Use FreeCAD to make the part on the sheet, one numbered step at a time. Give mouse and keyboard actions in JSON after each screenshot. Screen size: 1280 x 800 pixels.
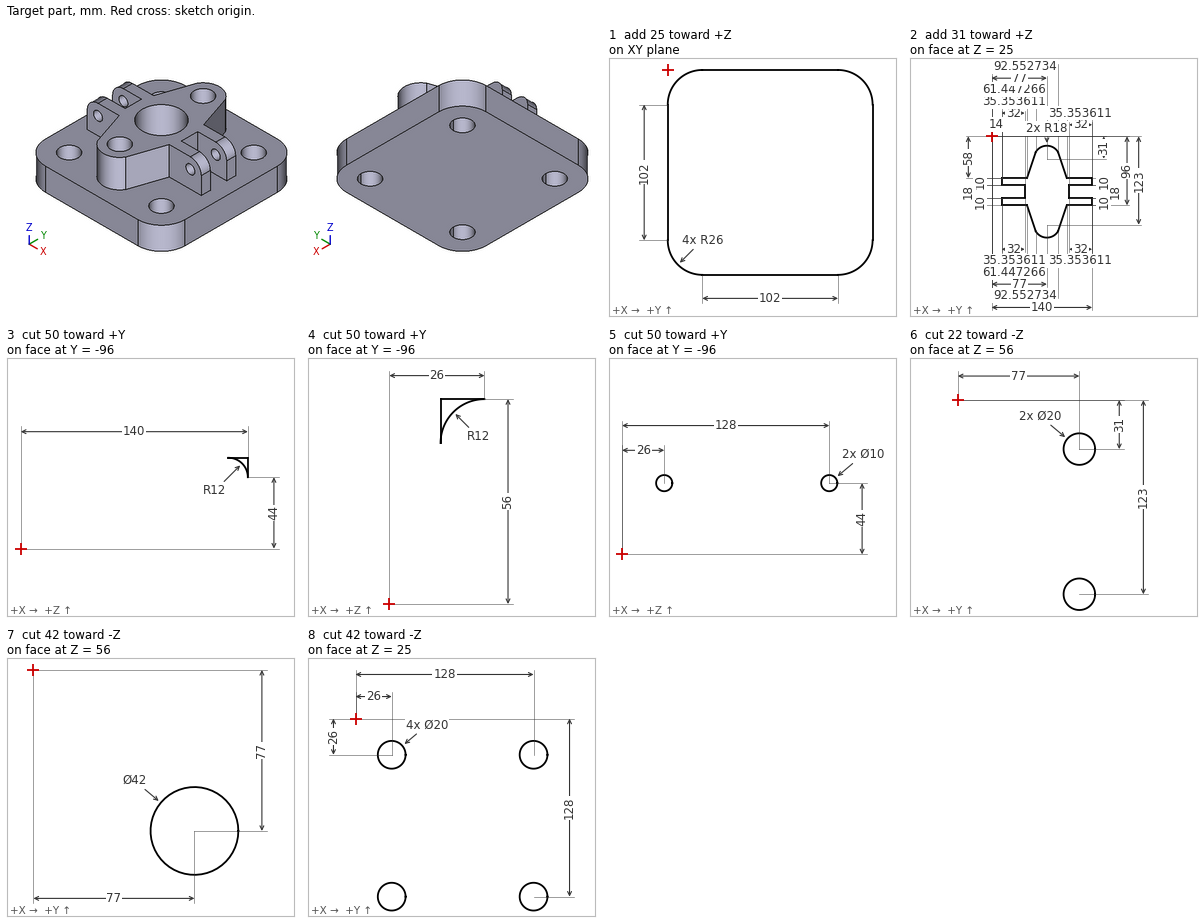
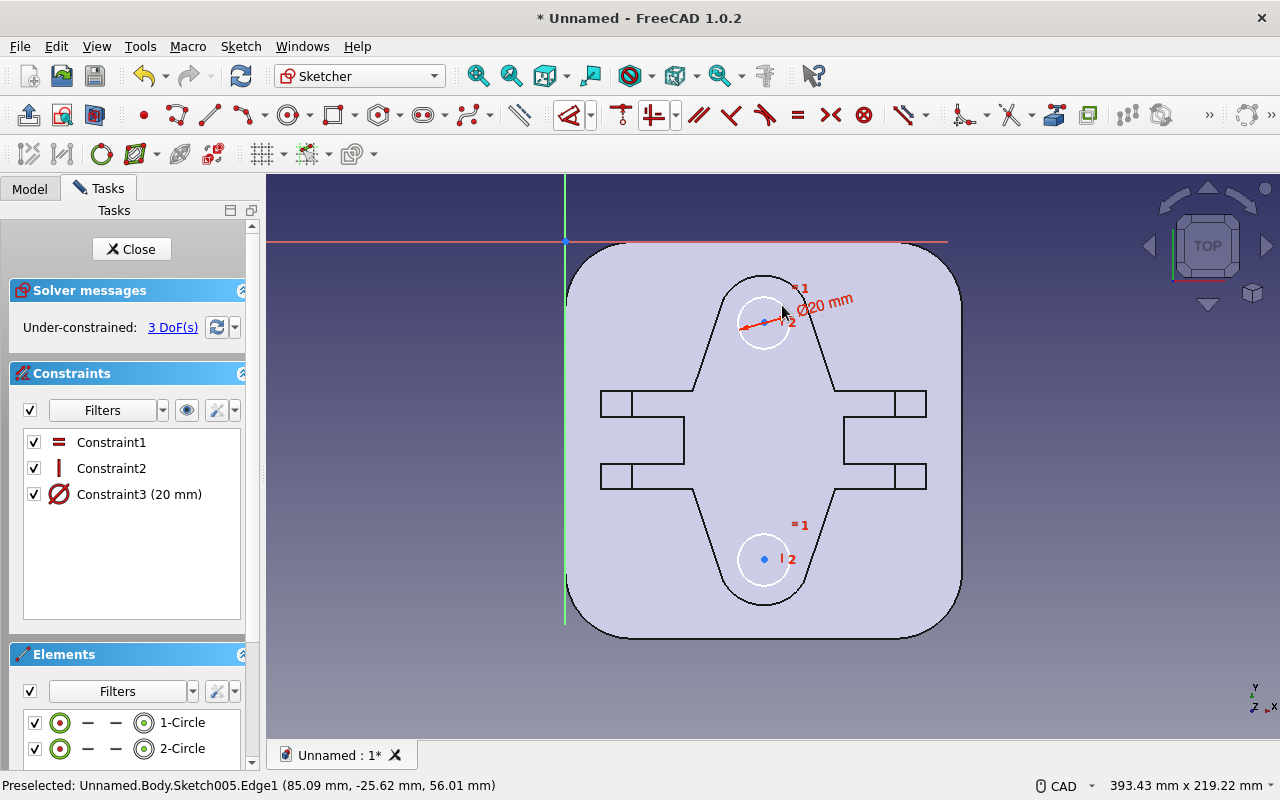
{"action": "left_click", "coordinate": [764, 323]}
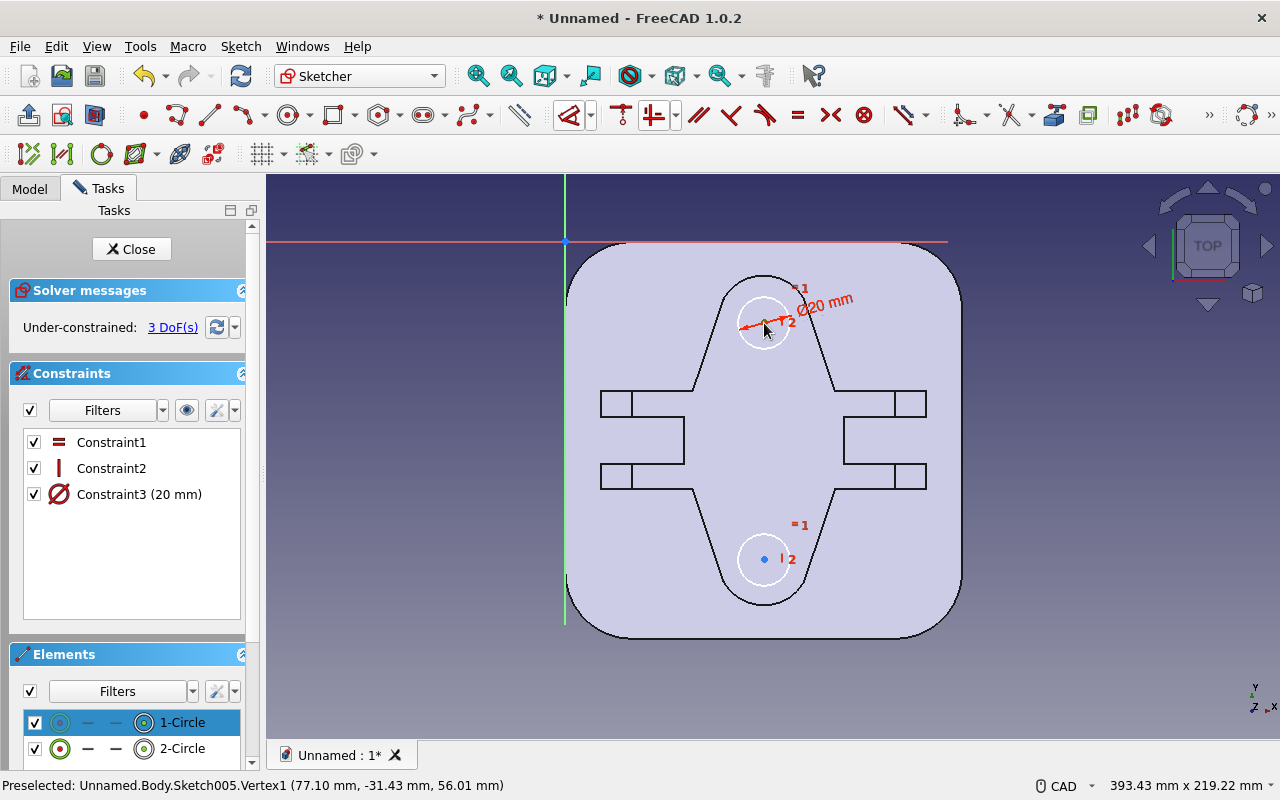
{"action": "left_click", "coordinate": [590, 116]}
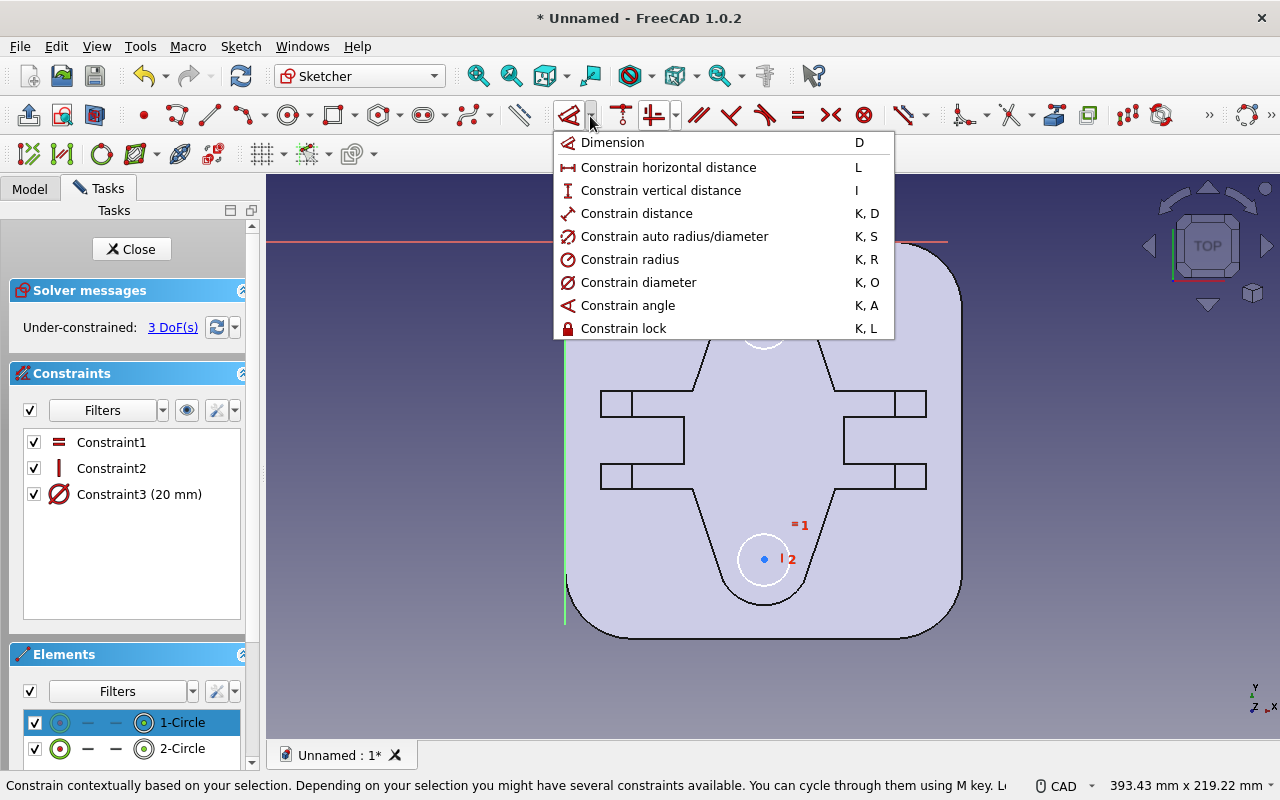
{"action": "left_click", "coordinate": [724, 168]}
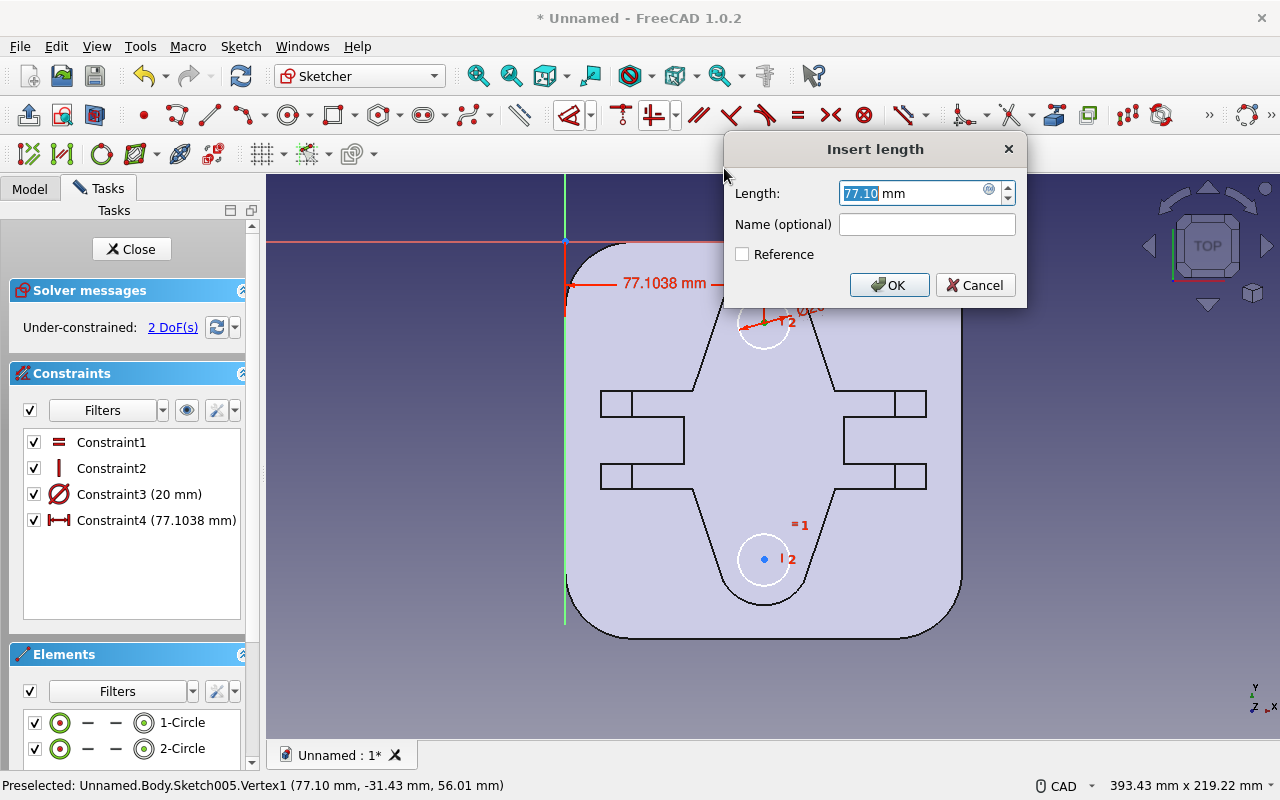
{"action": "type", "text": "77"}
{"action": "key", "text": "Return"}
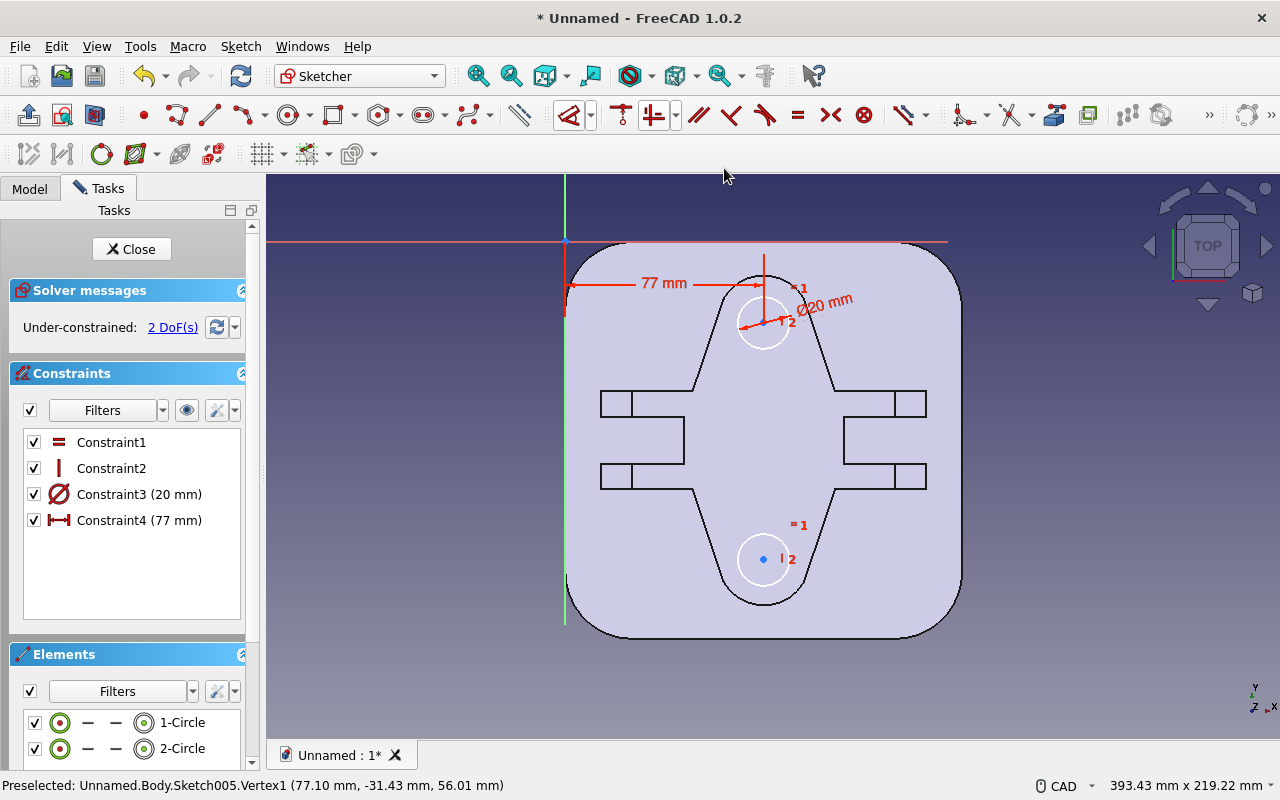
{"action": "left_click", "coordinate": [764, 323]}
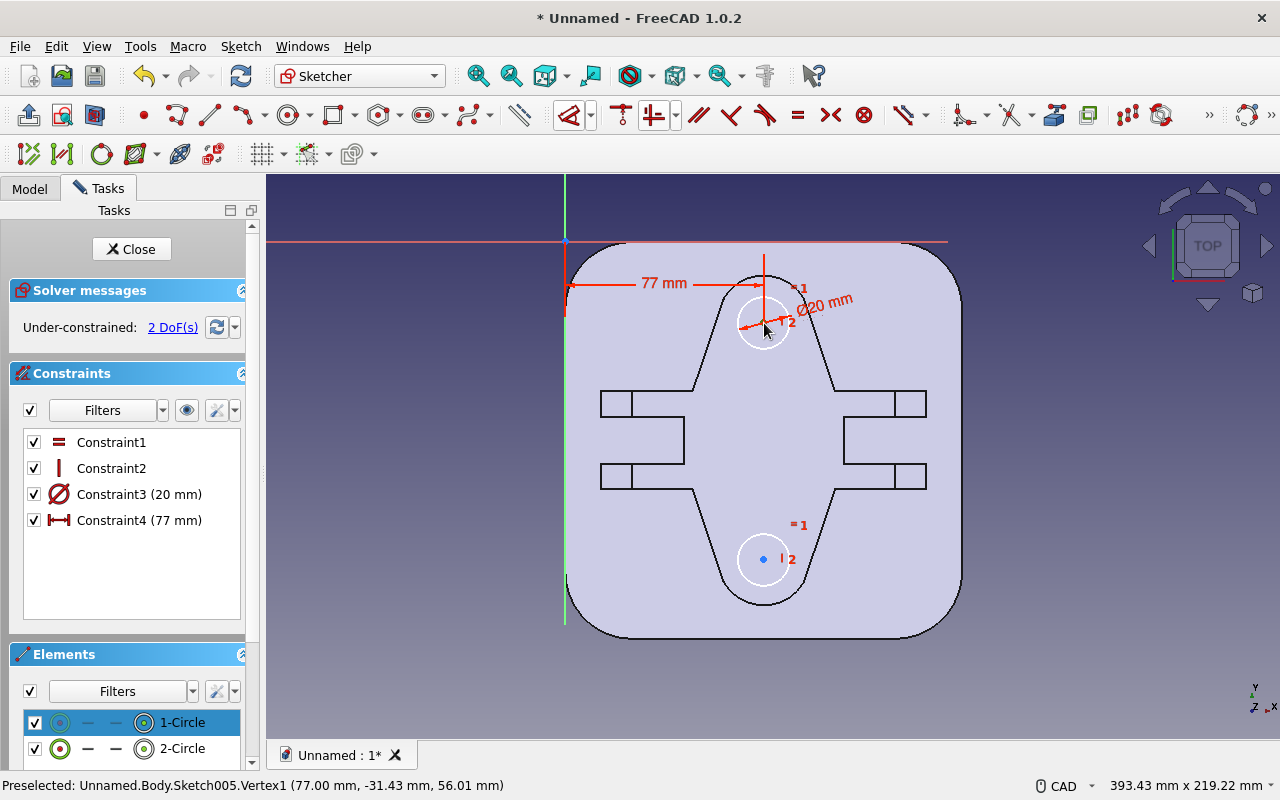
{"action": "key", "text": "i"}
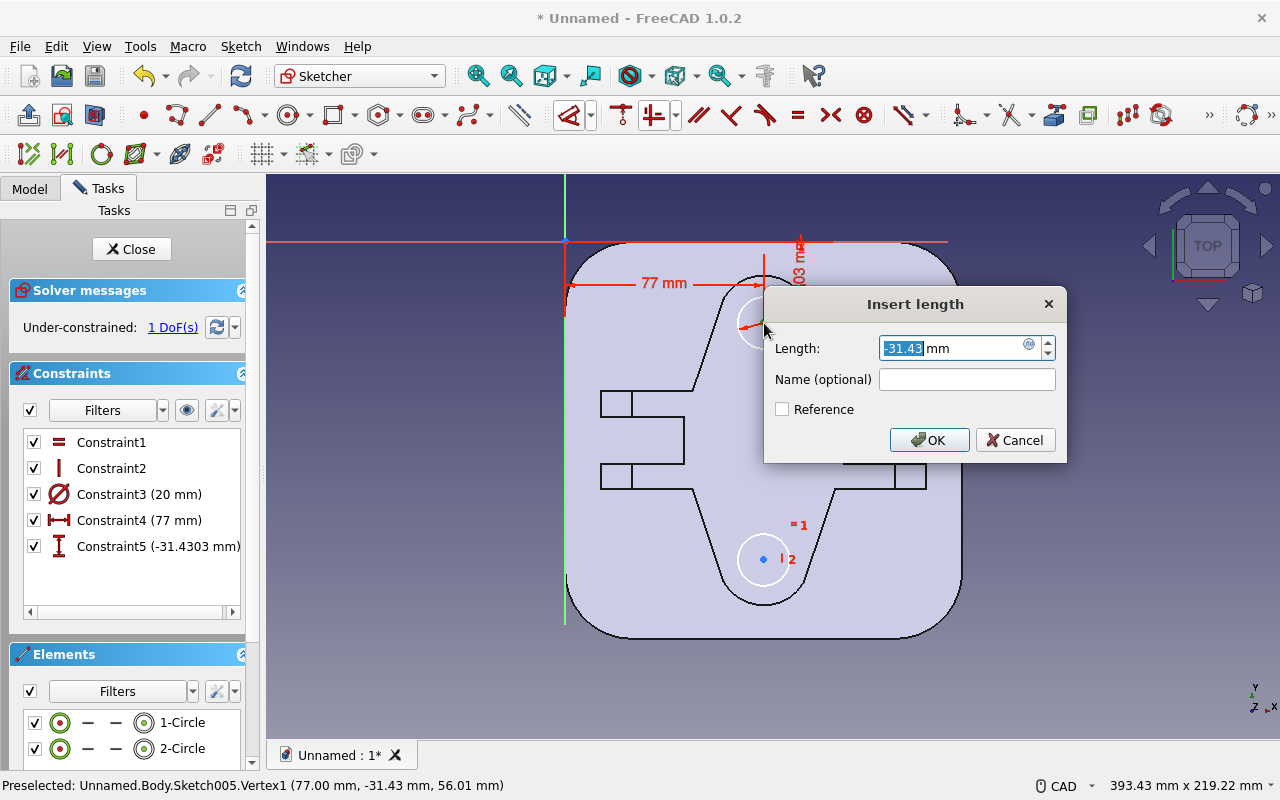
{"action": "type", "text": "-31"}
{"action": "key", "text": "Return"}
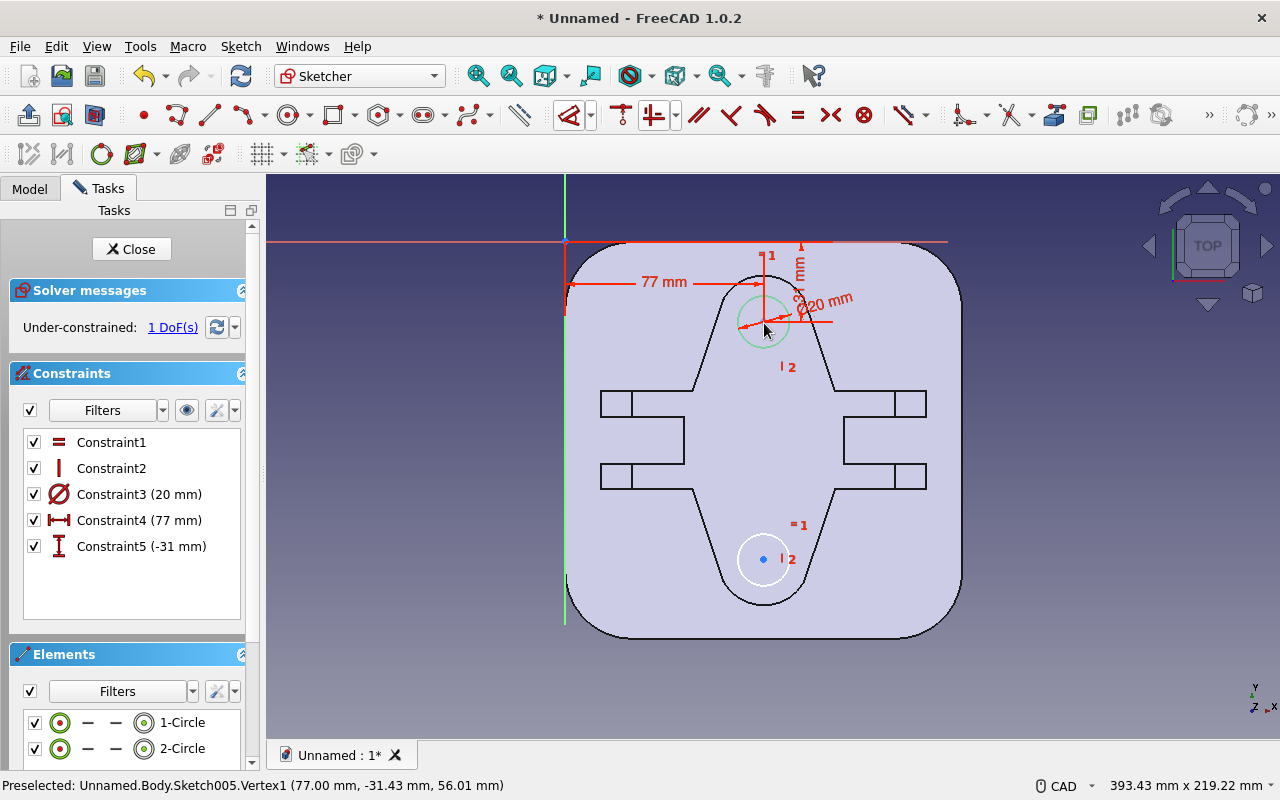
{"action": "left_click", "coordinate": [764, 560]}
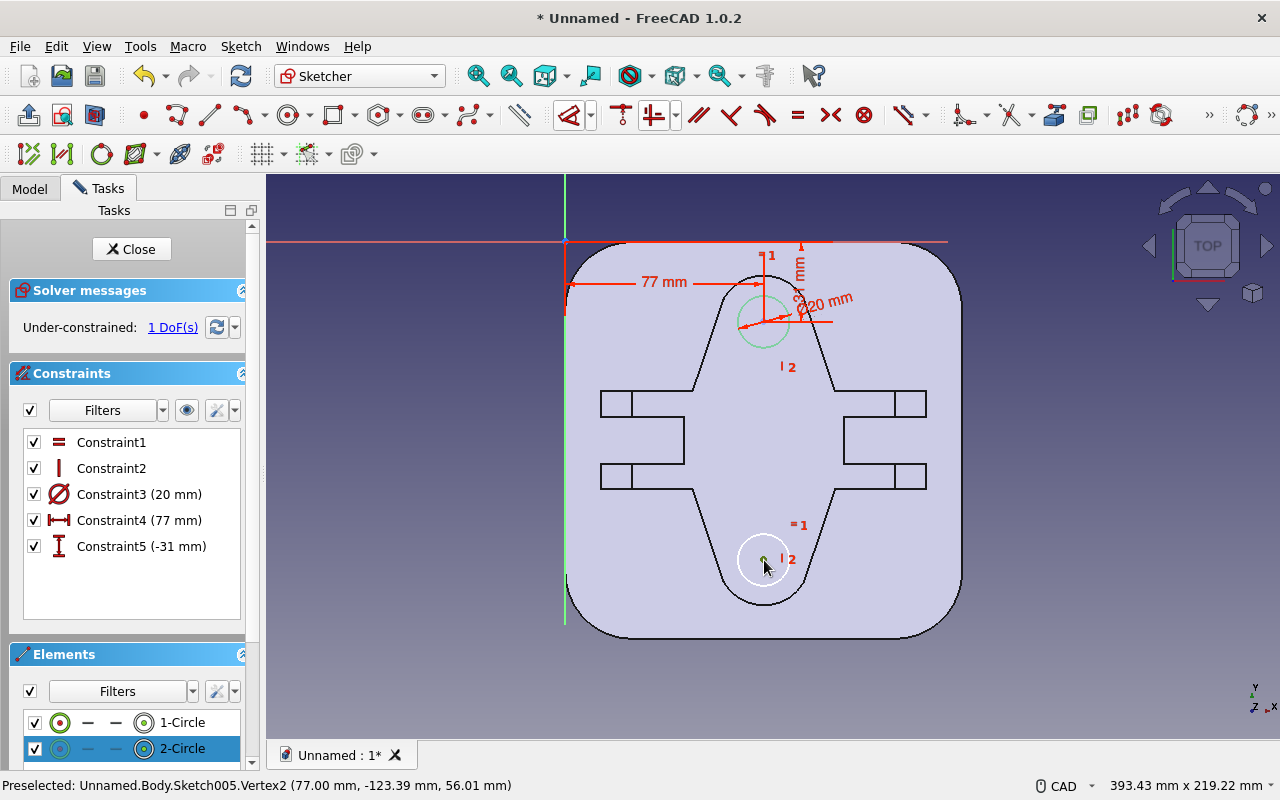
{"action": "key", "text": "i"}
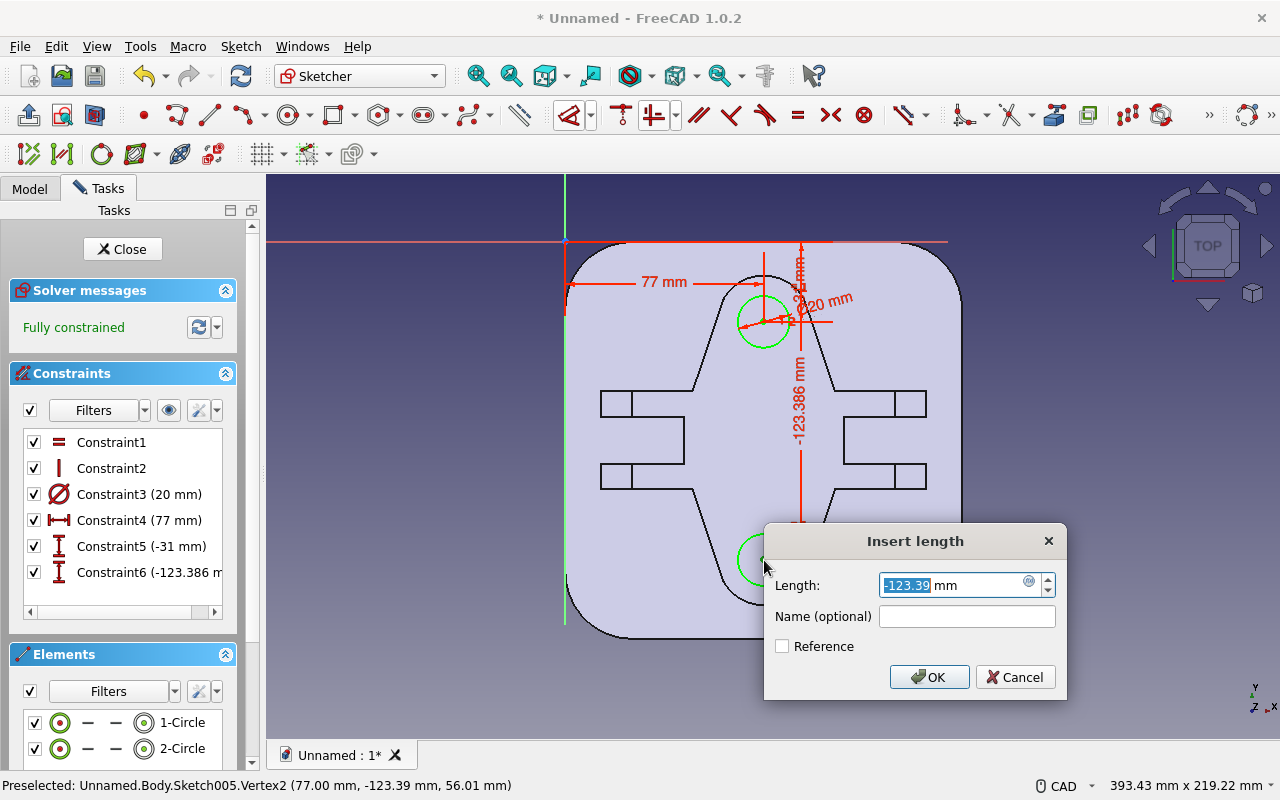
{"action": "type", "text": "-123"}
{"action": "key", "text": "Return"}